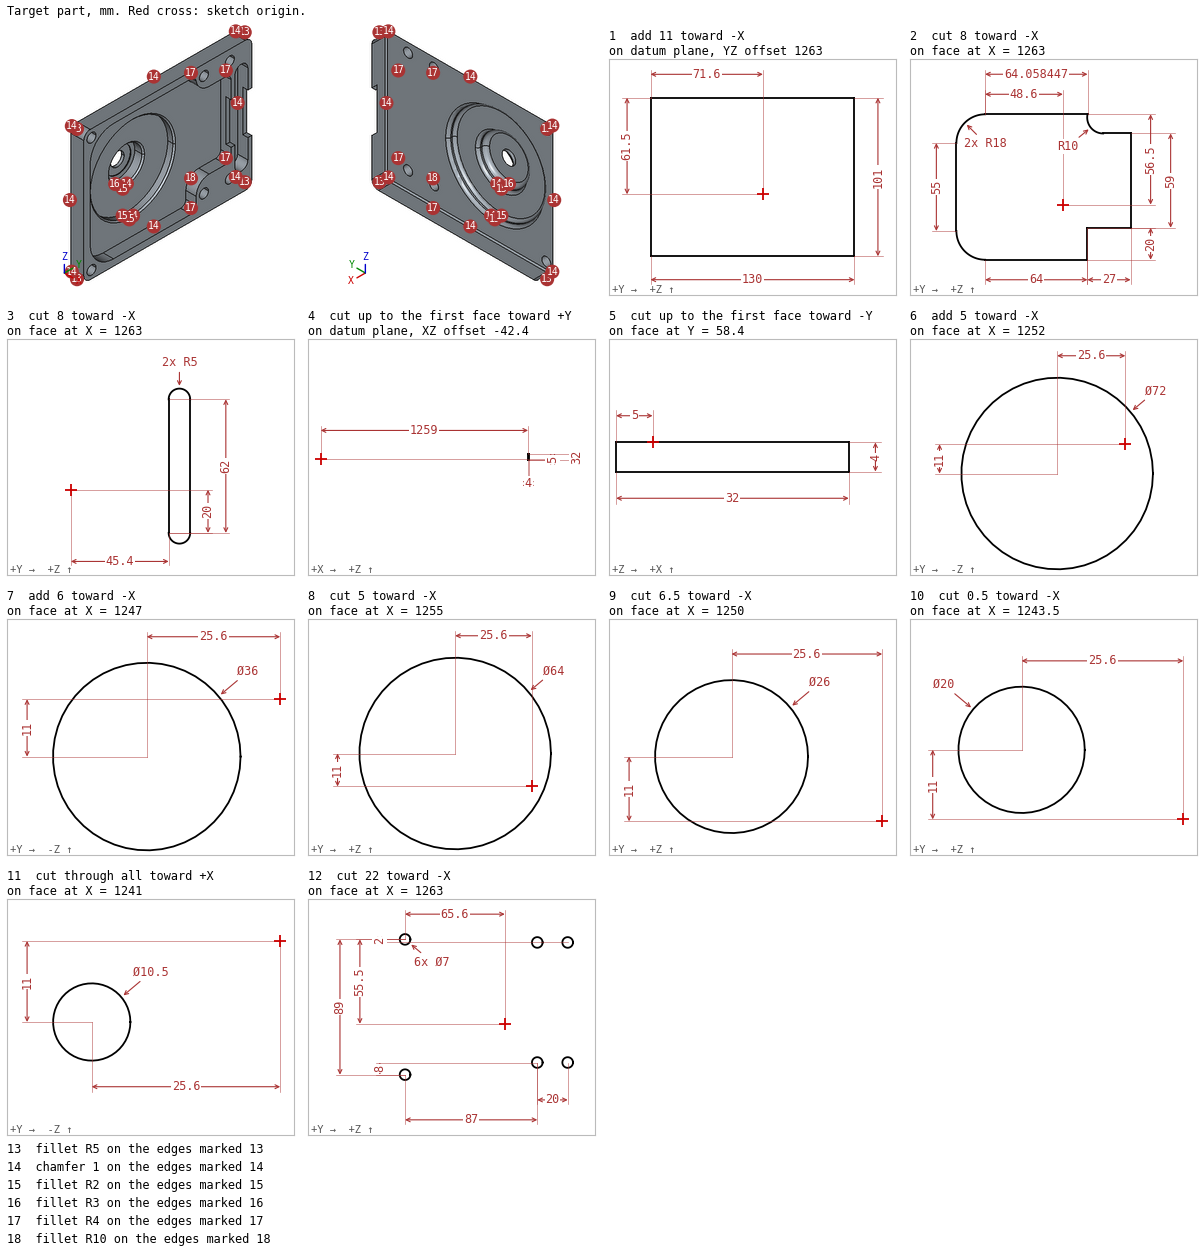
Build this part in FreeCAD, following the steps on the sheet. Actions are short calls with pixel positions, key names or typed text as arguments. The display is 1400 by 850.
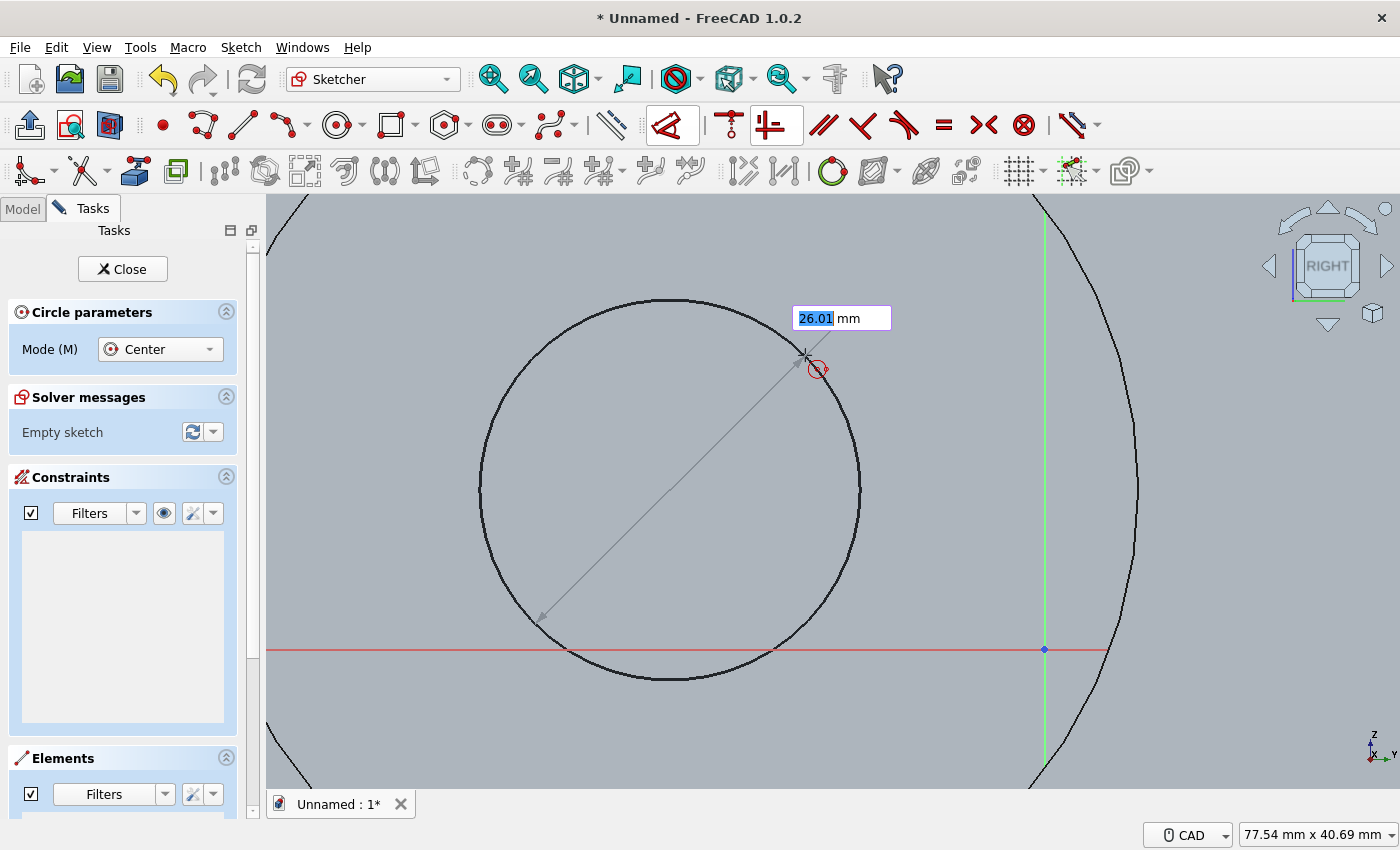
text(26)
key(Return)
key(Escape)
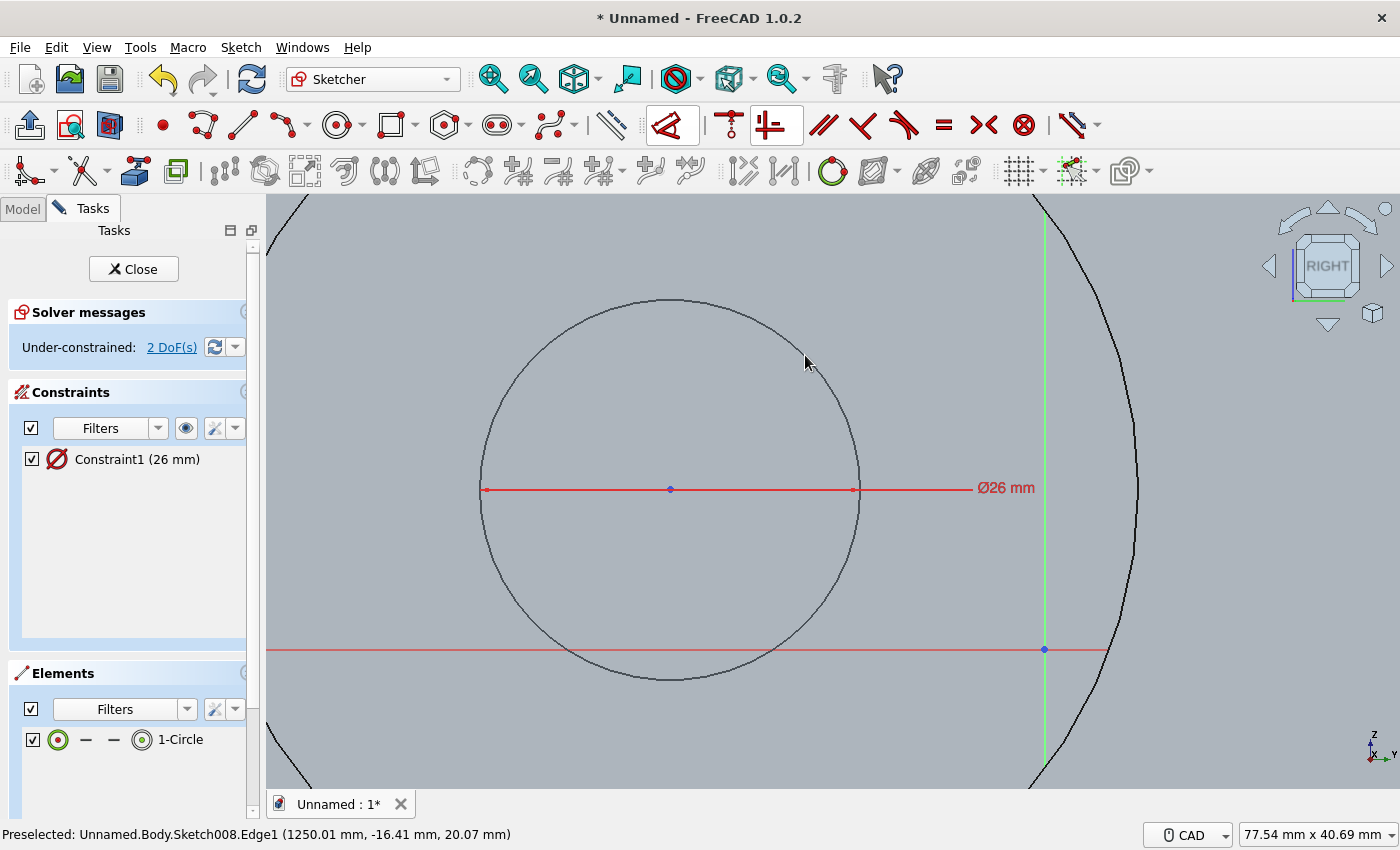
click(670, 490)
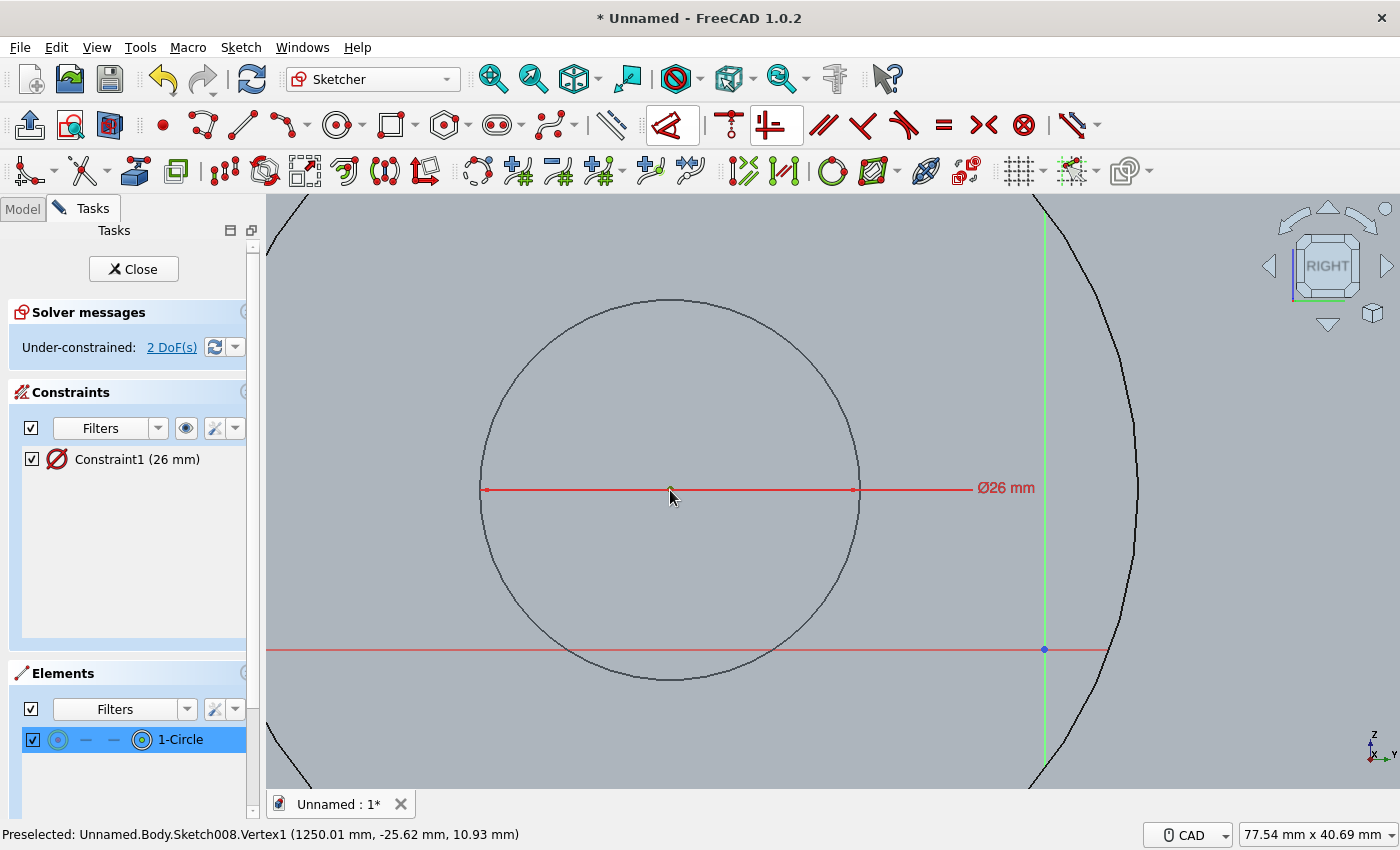
key(i)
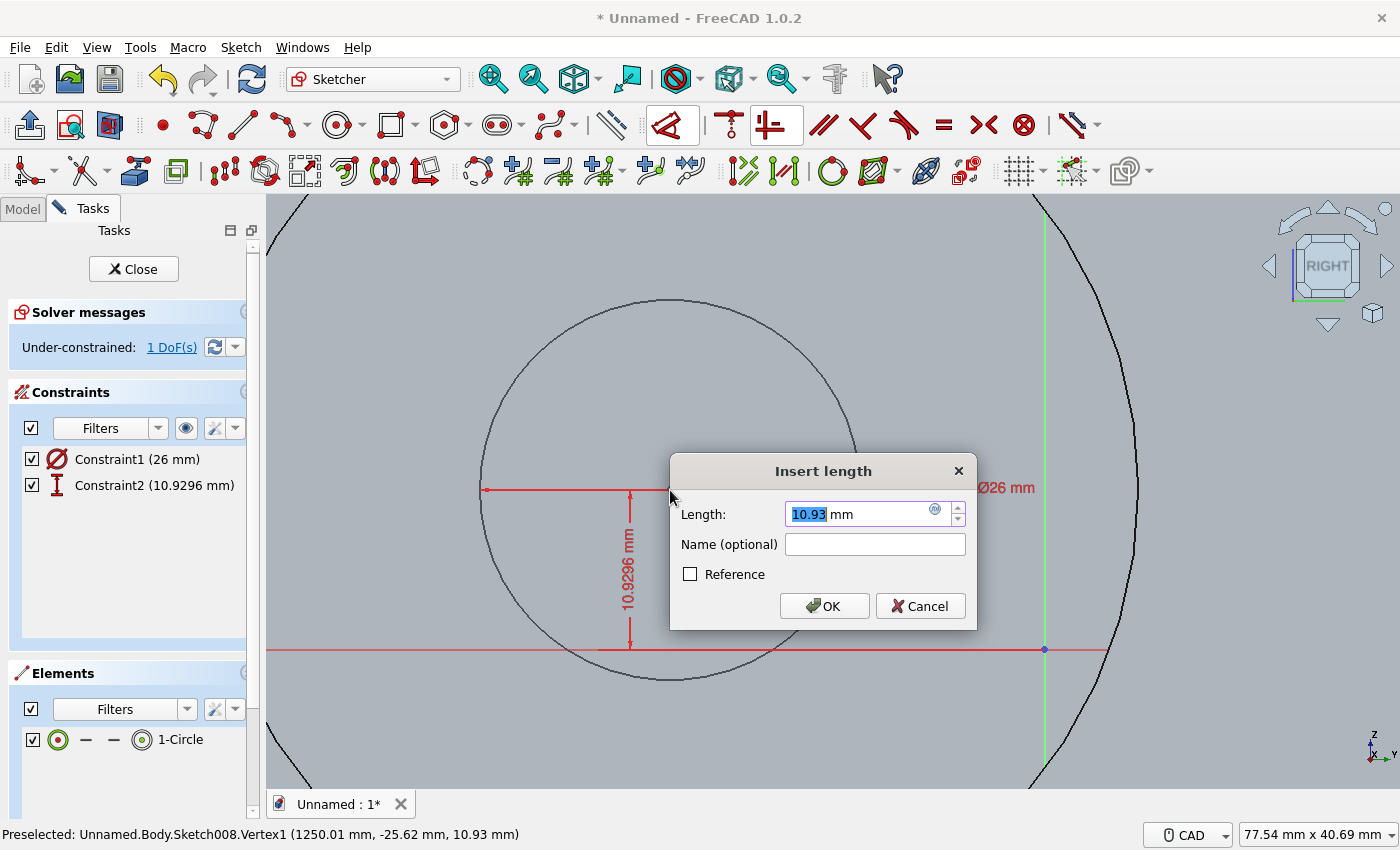
text(11)
key(Return)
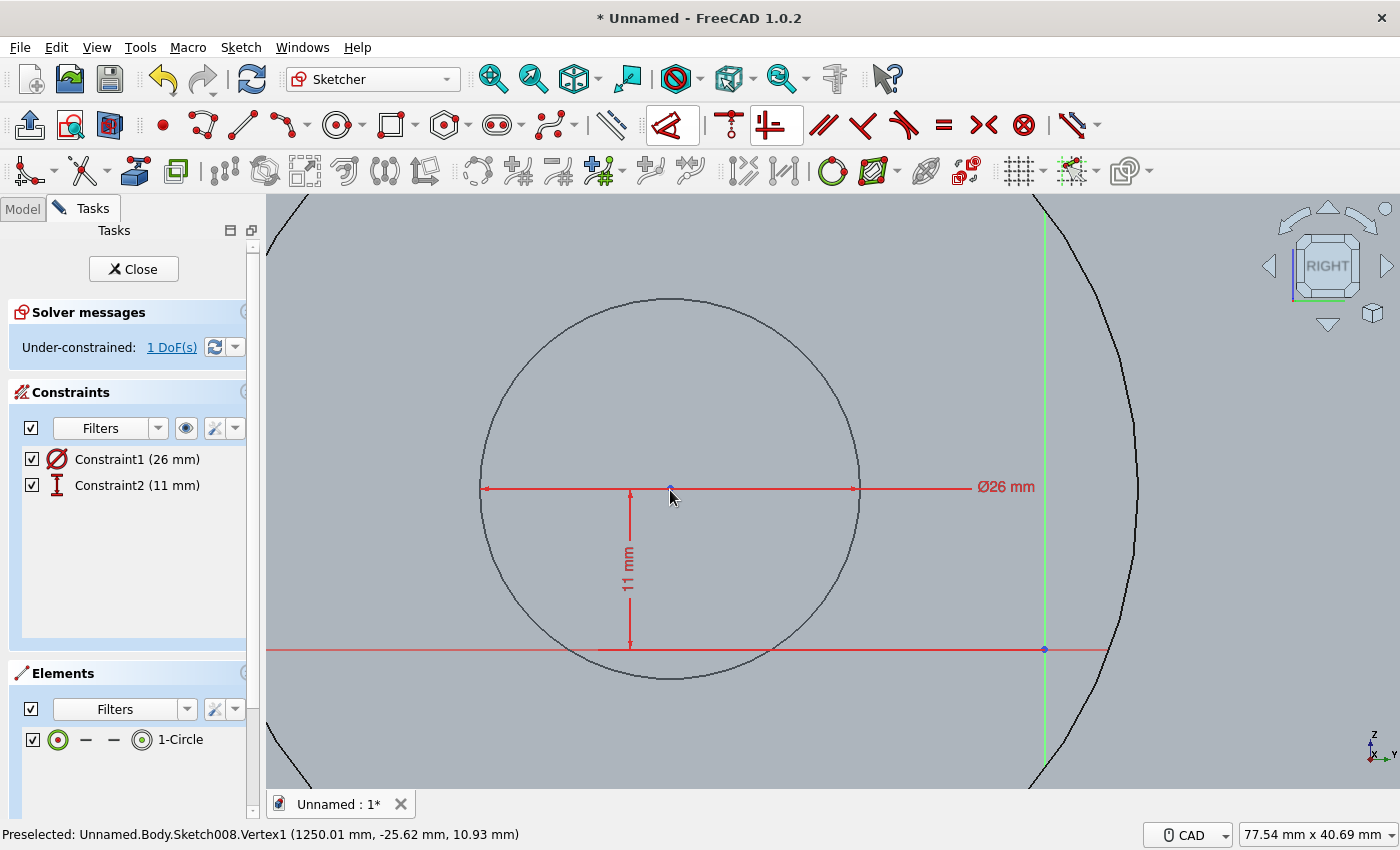
click(670, 489)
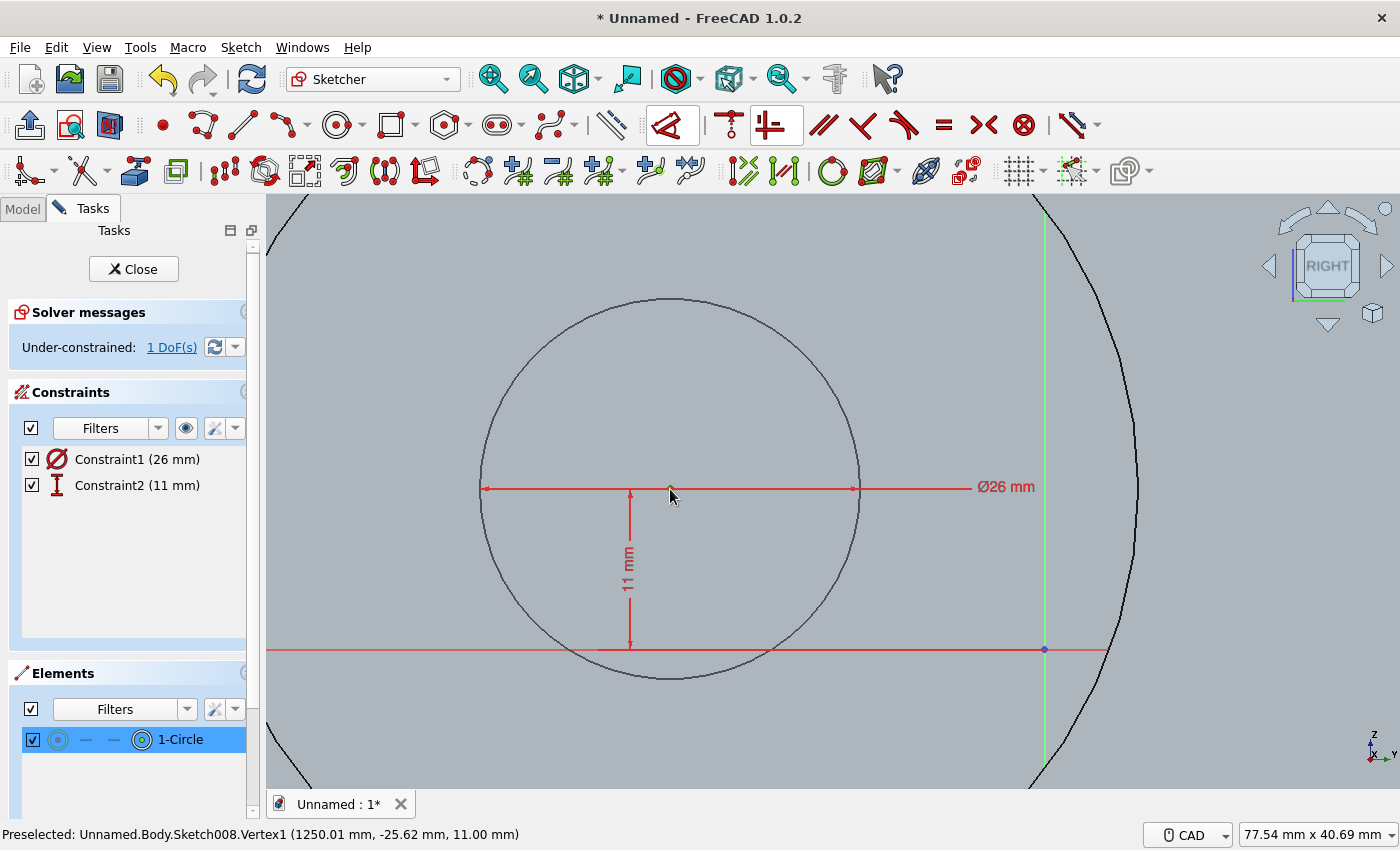
key(l)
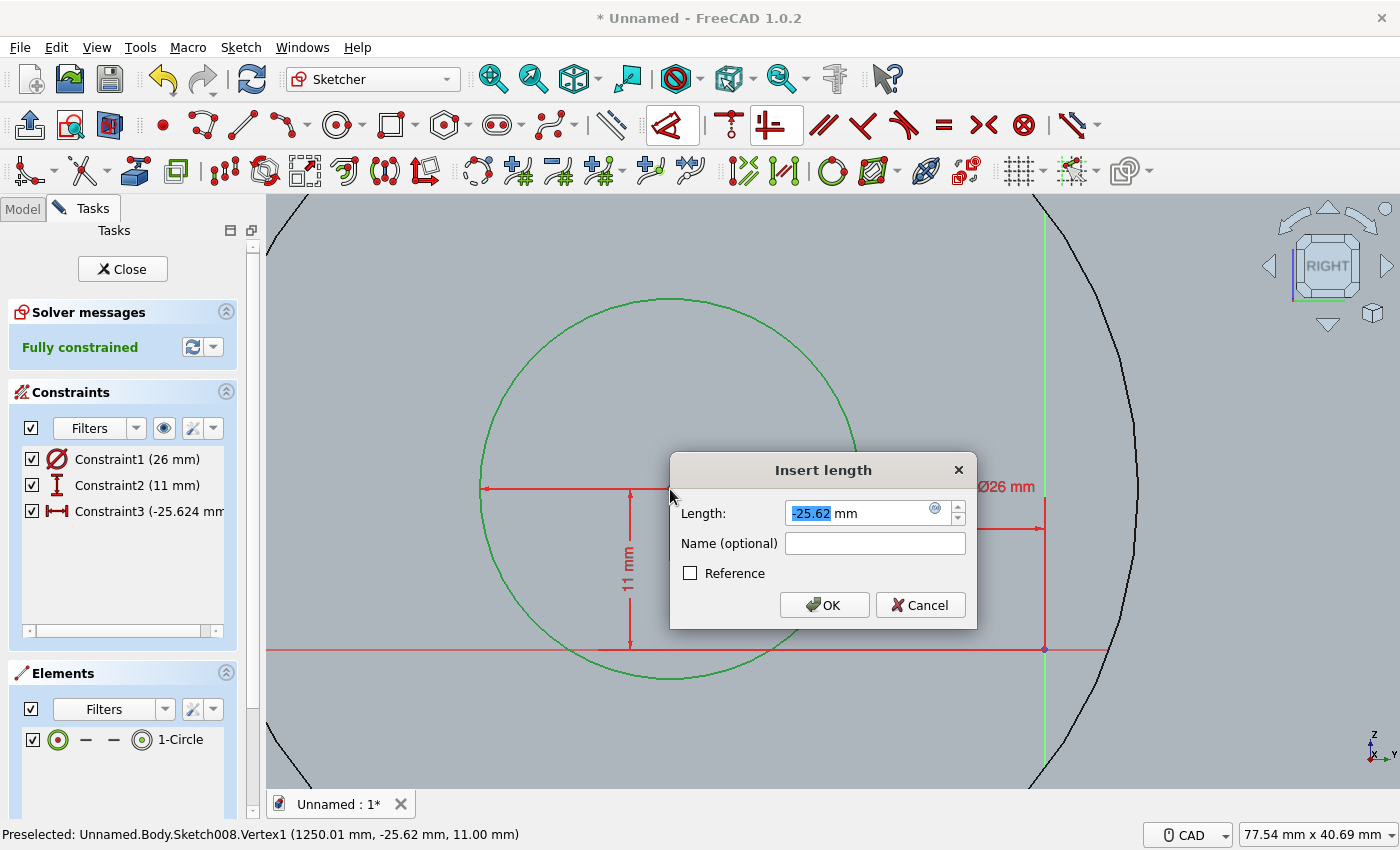
text(-25.6)
key(Return)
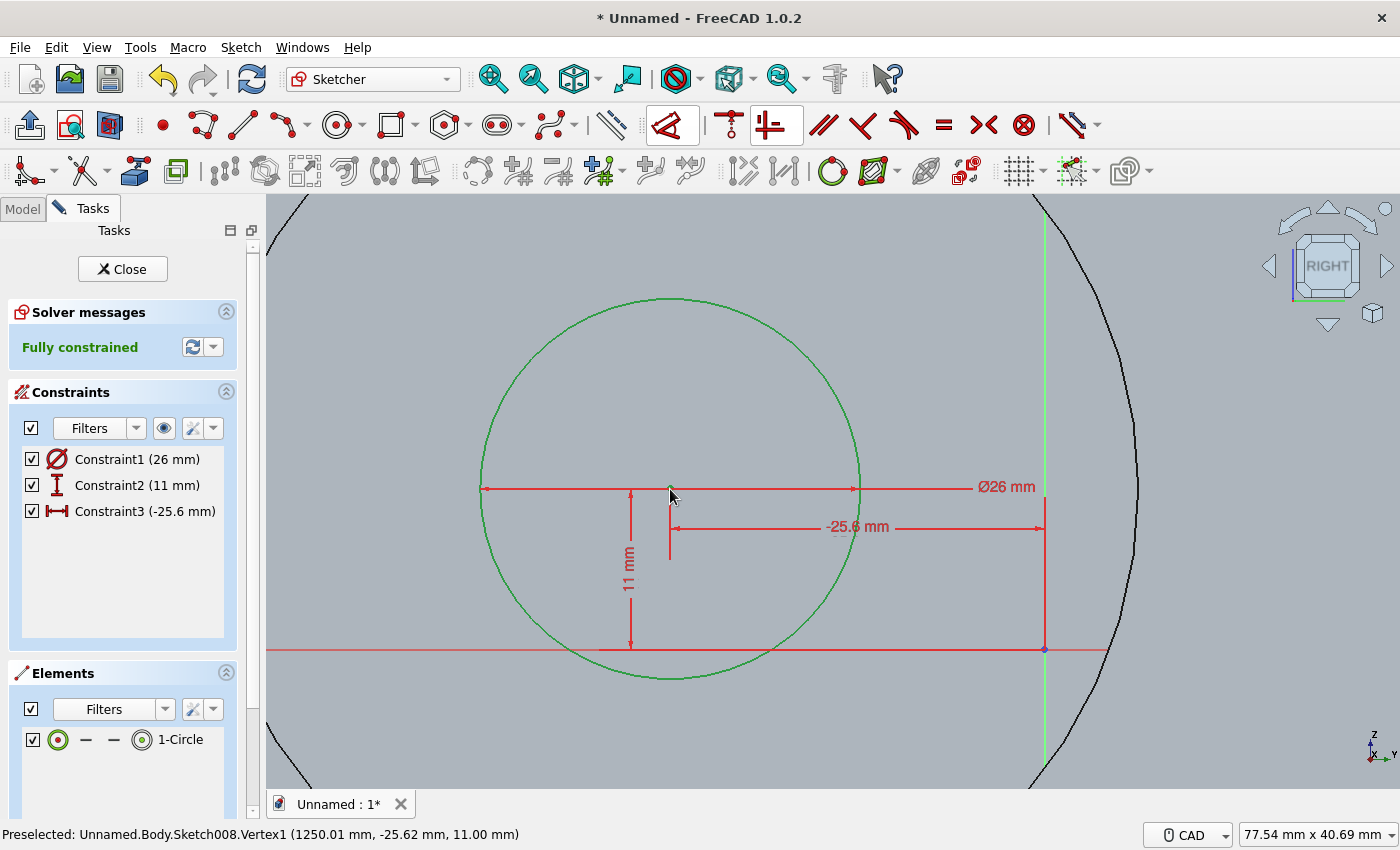
click(123, 269)